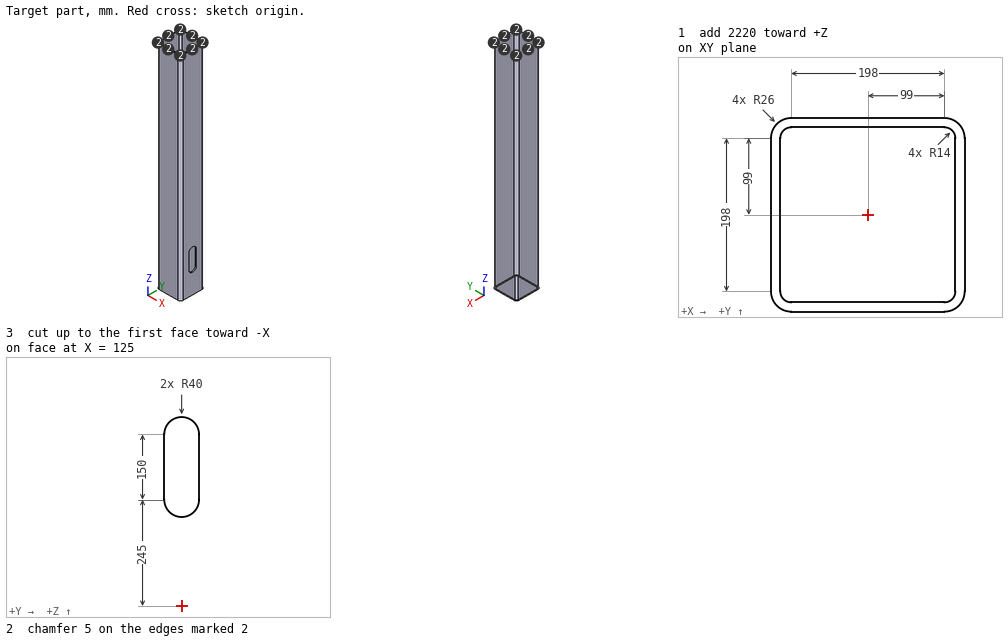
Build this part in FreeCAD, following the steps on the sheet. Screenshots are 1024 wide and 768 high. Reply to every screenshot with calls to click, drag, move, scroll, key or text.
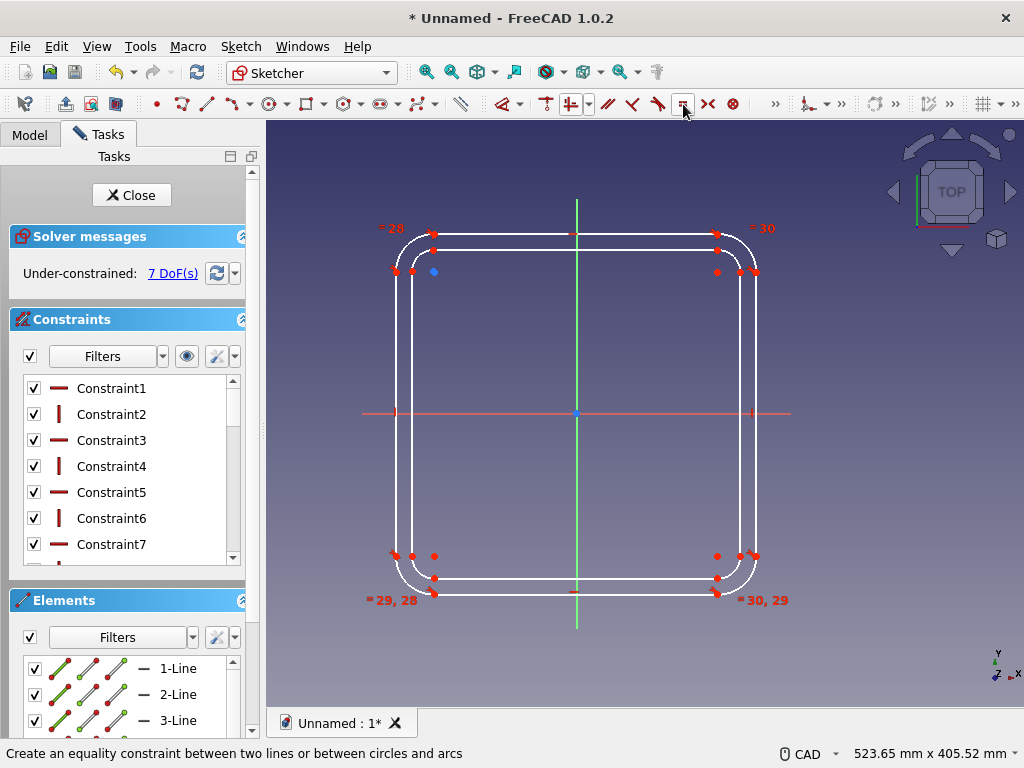
scroll(738, 262, up, 2)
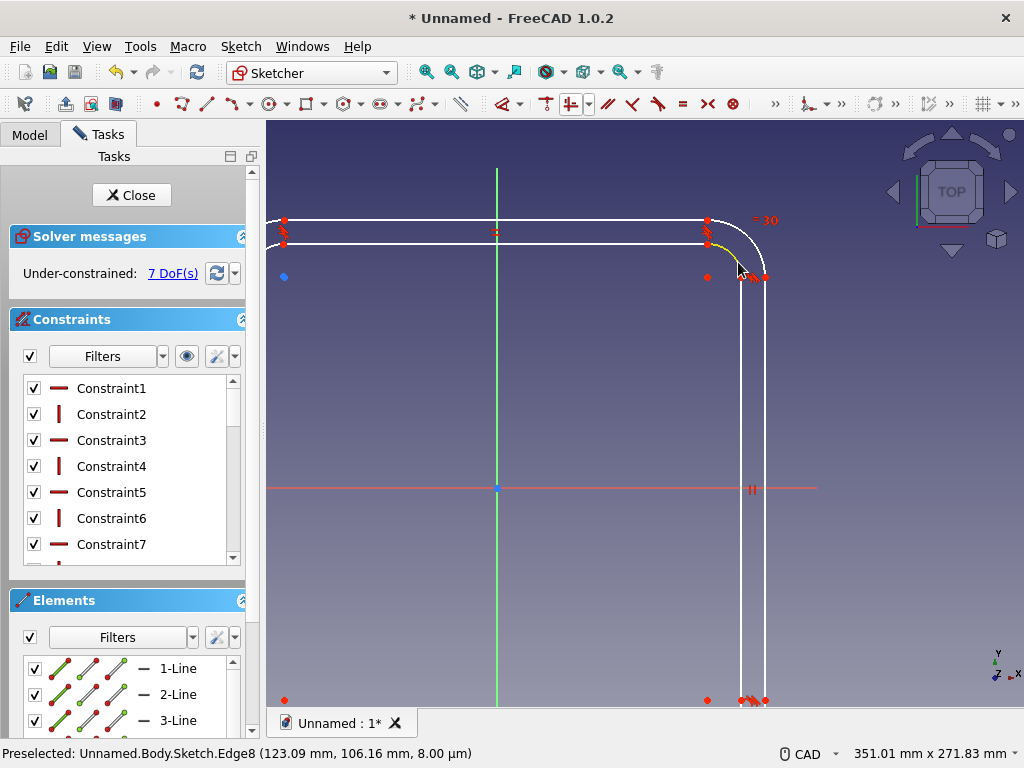
click(737, 262)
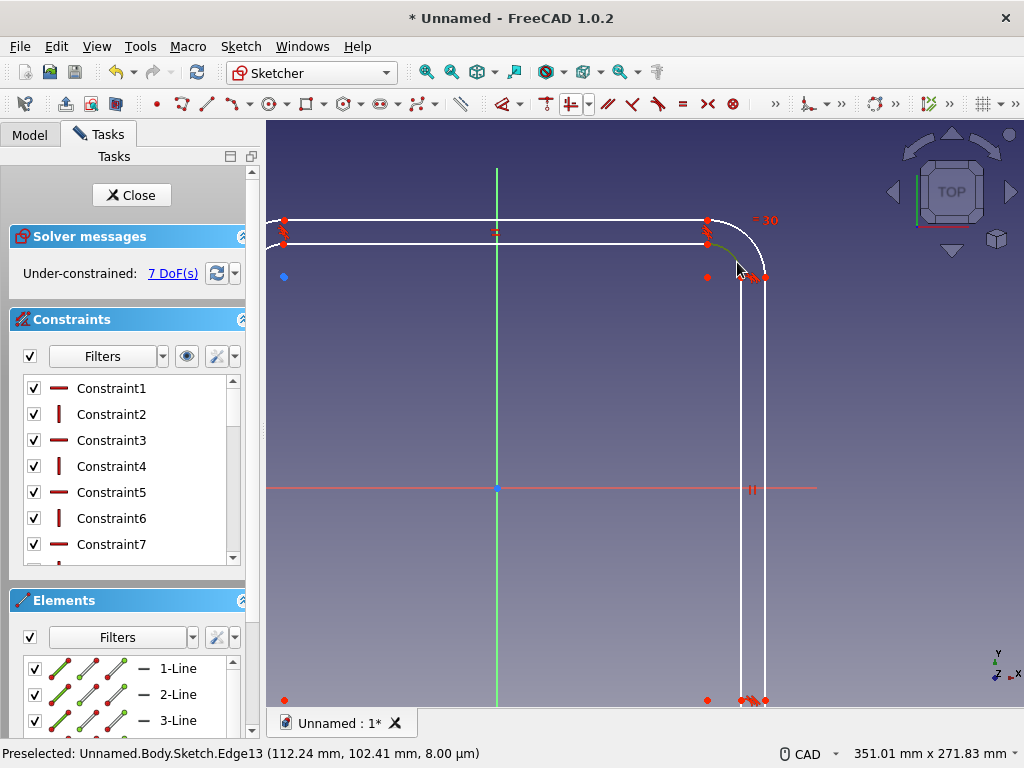
scroll(738, 262, down, 2)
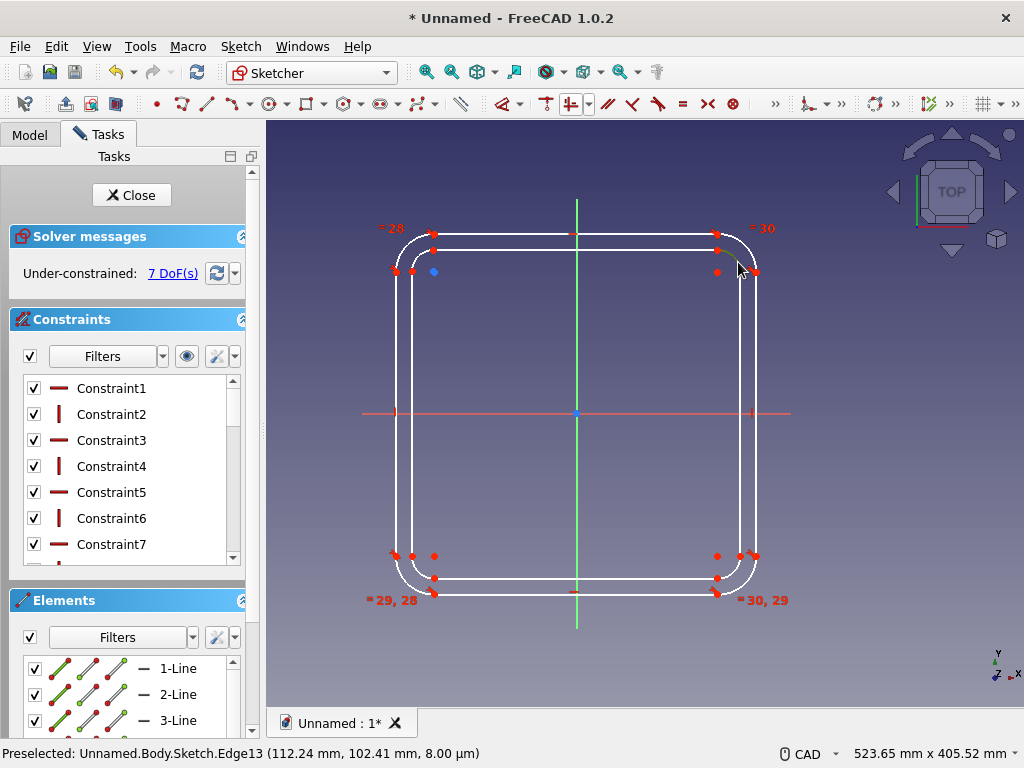
scroll(424, 252, up, 2)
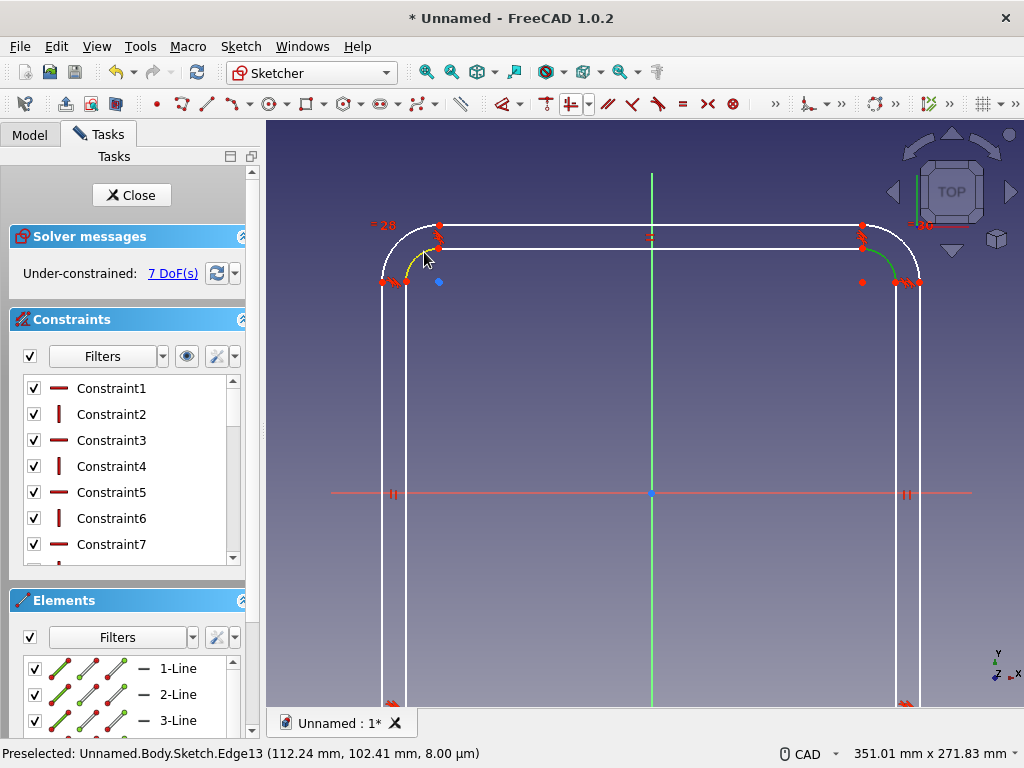
click(424, 252)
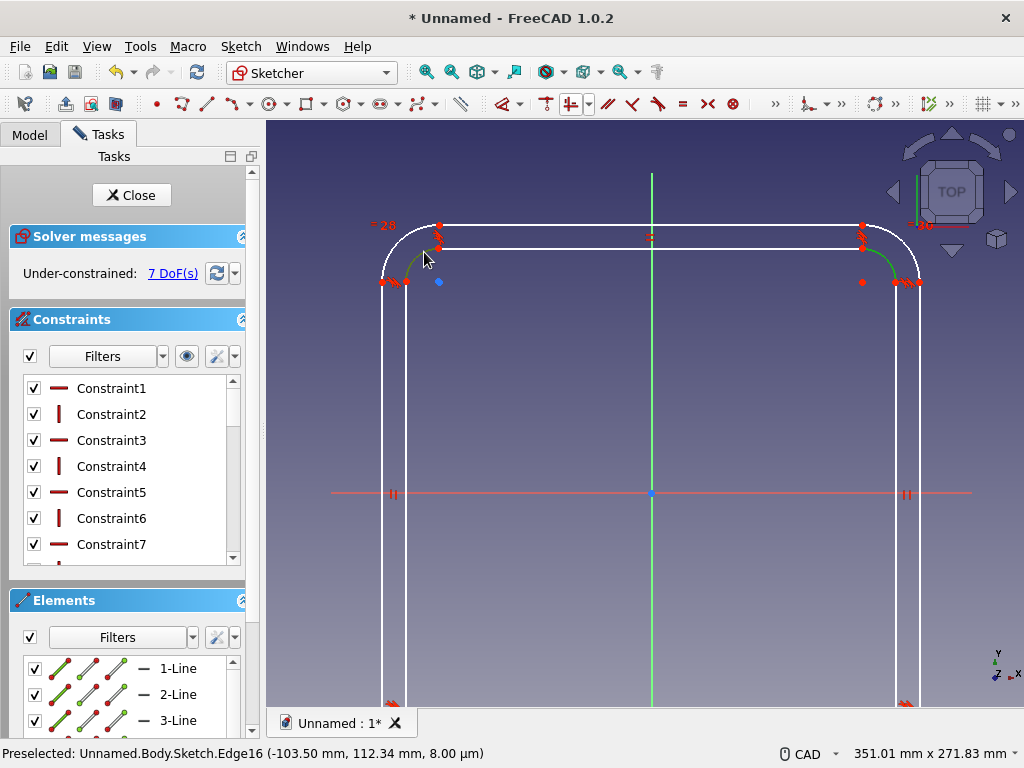
click(683, 104)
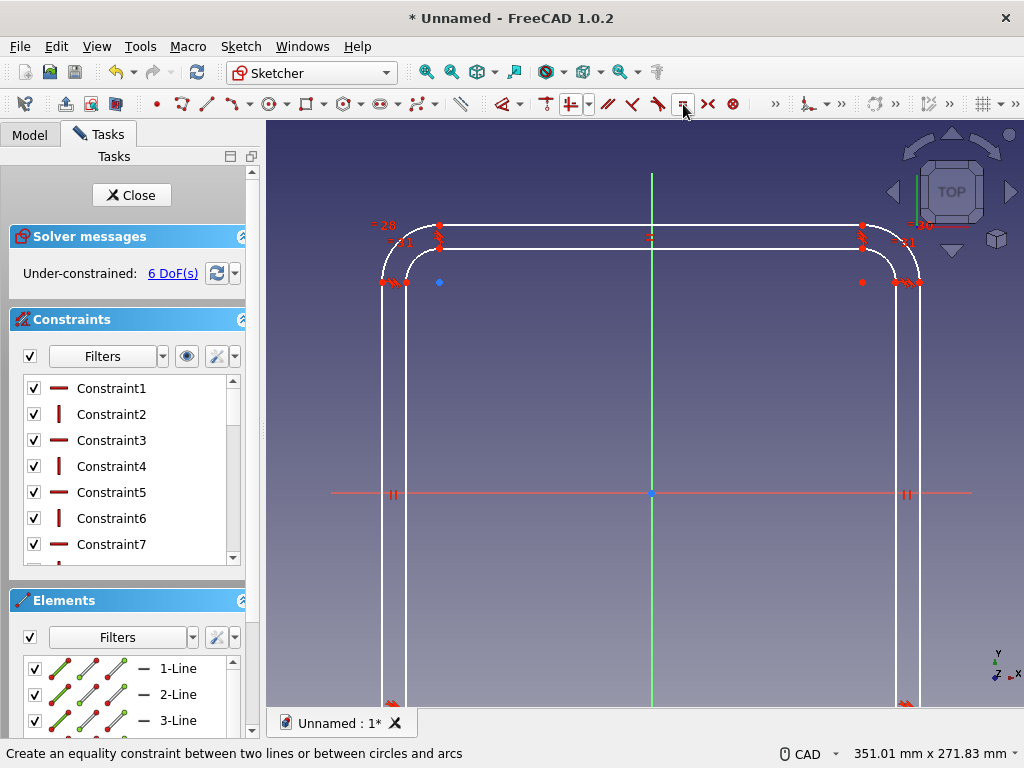
click(502, 104)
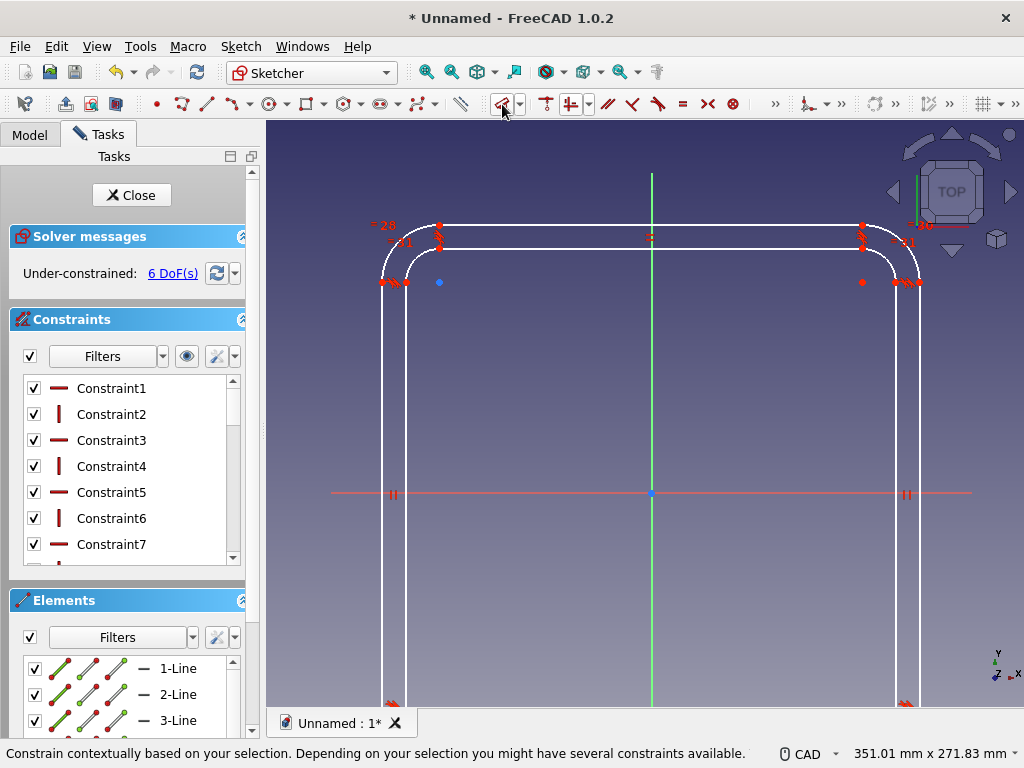
click(413, 231)
click(398, 203)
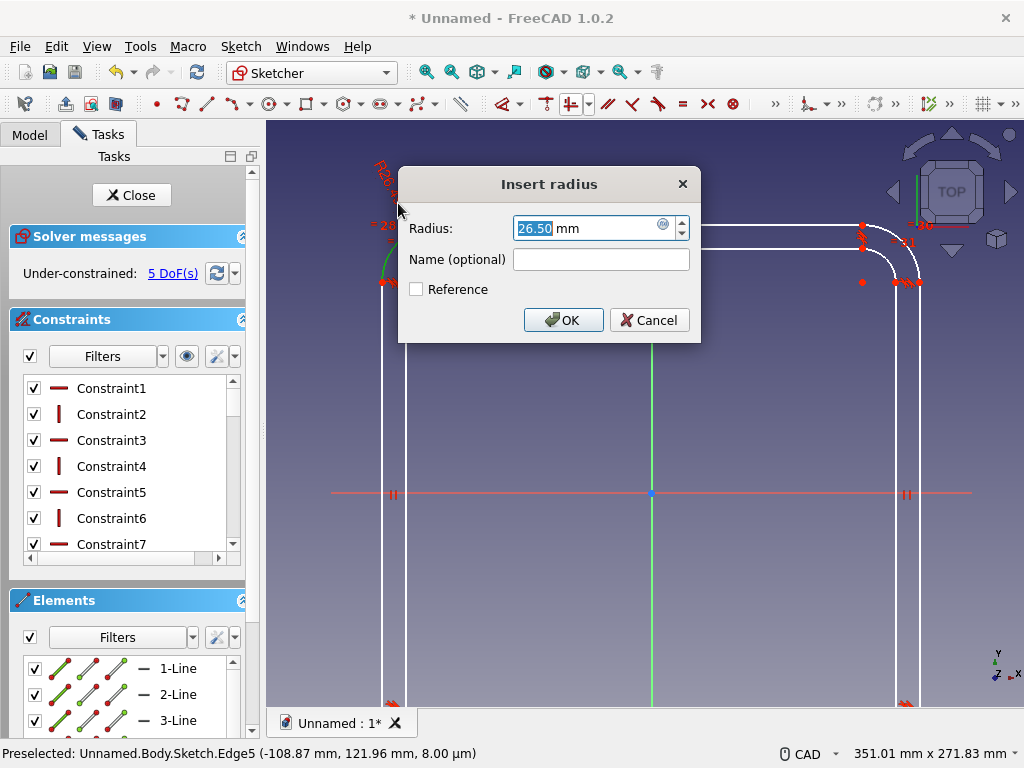
text(26)
key(Return)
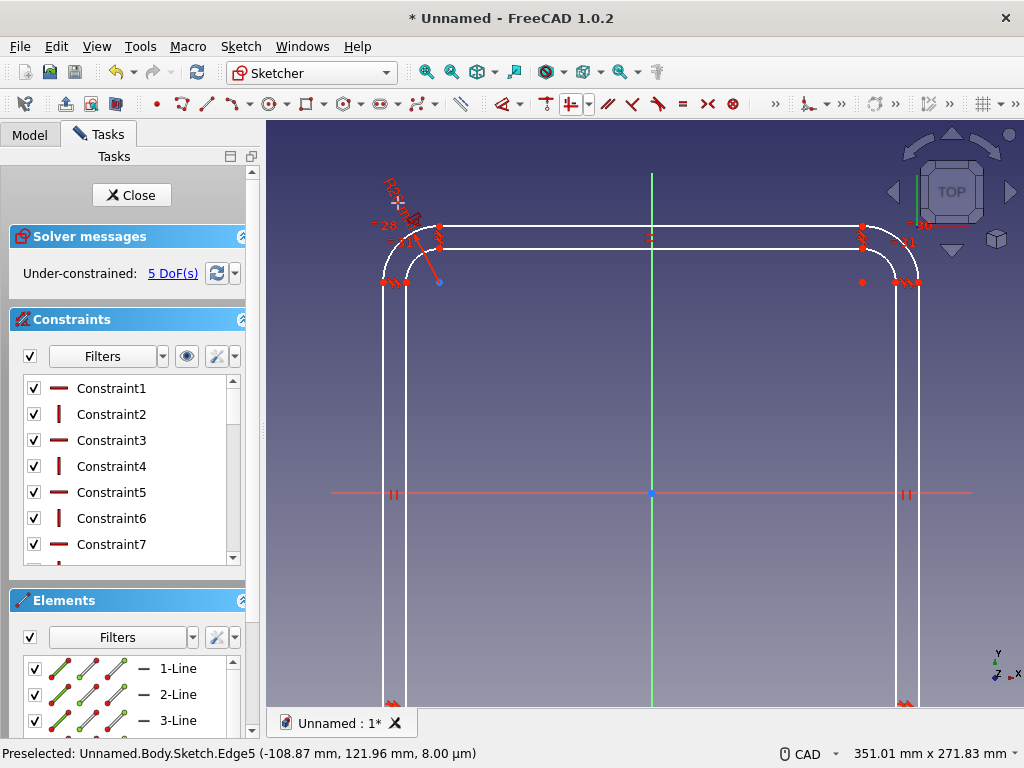
scroll(424, 252, down, 2)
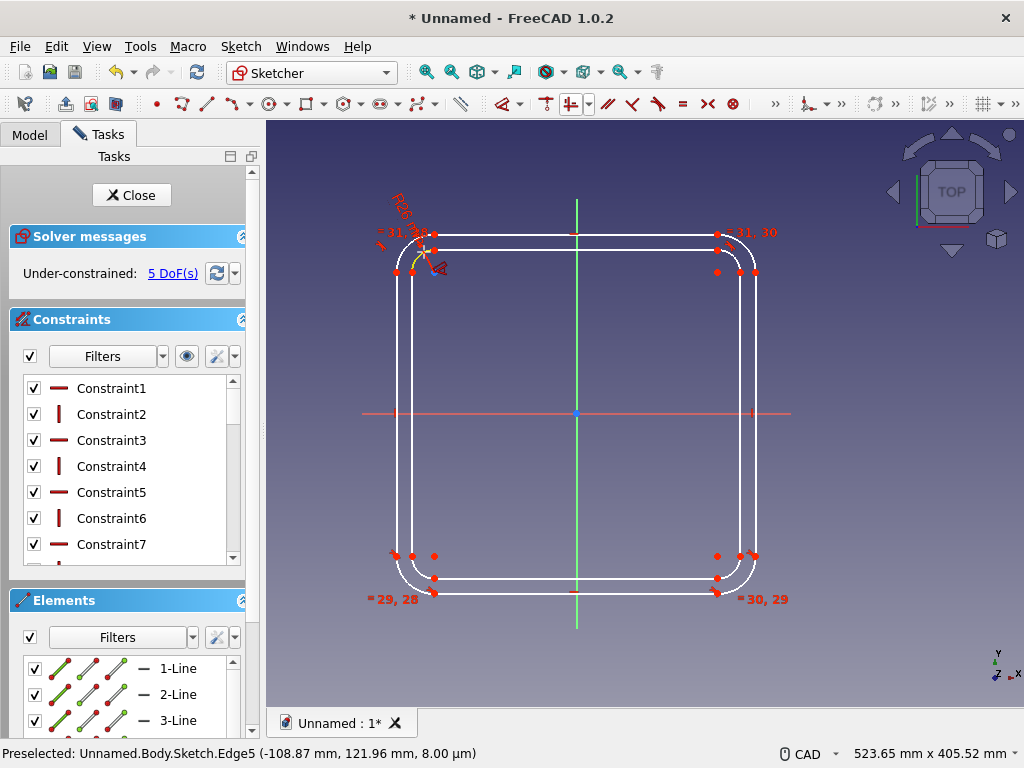
scroll(738, 262, up, 4)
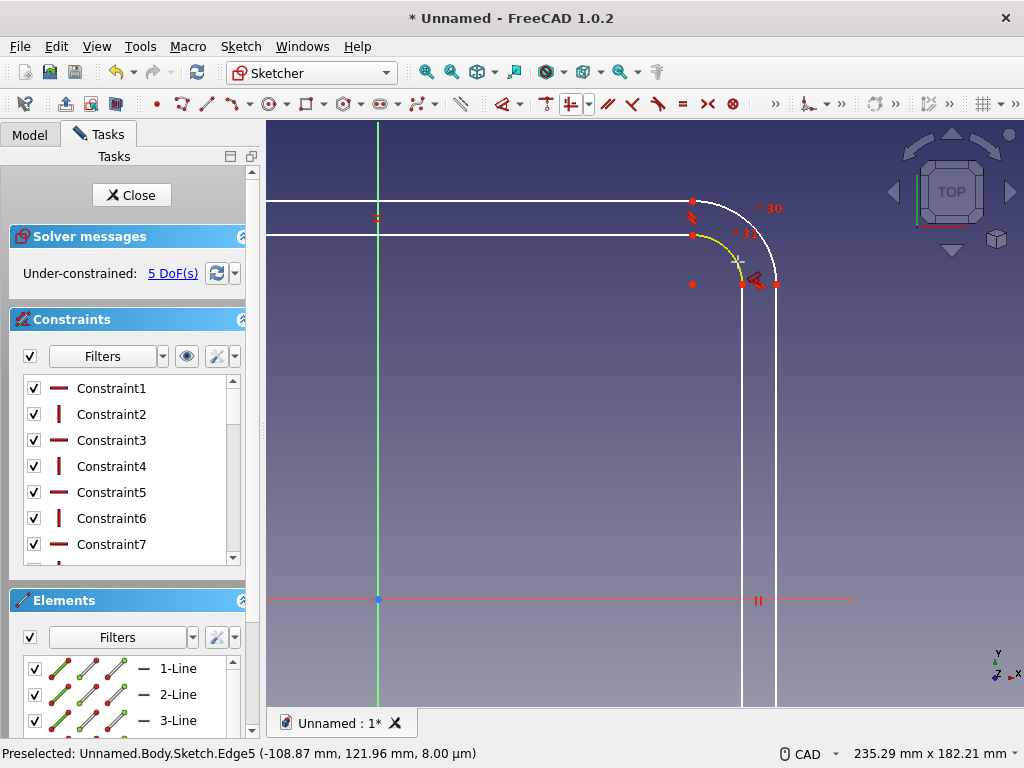
click(737, 262)
click(620, 322)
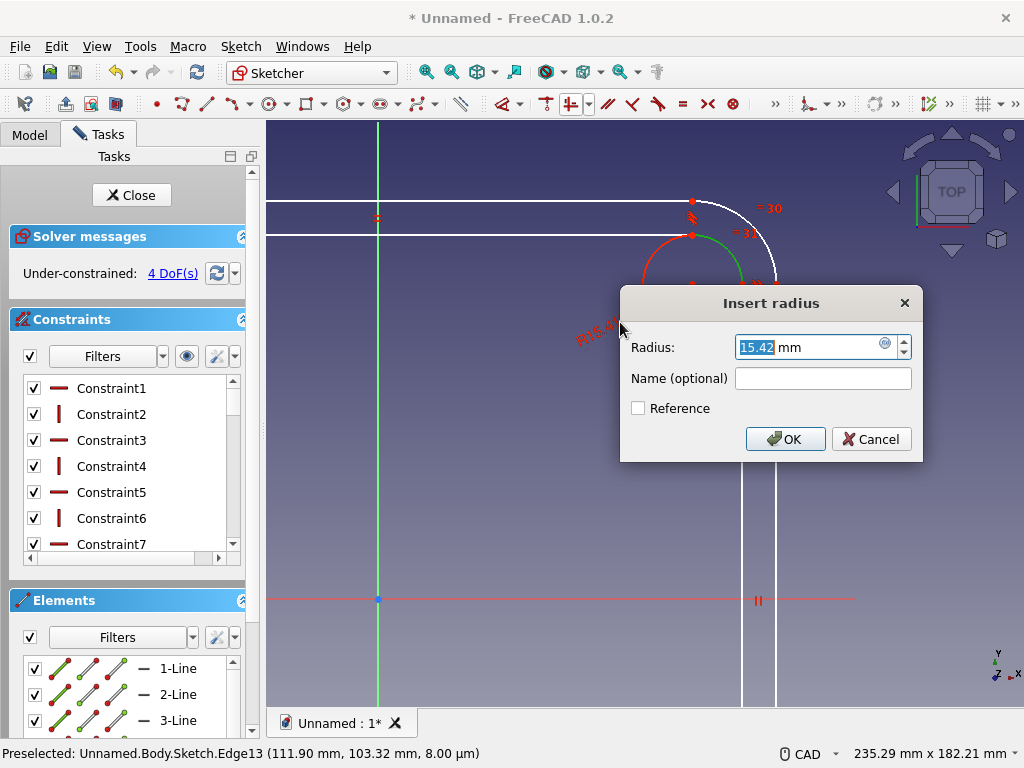
text(14)
key(Return)